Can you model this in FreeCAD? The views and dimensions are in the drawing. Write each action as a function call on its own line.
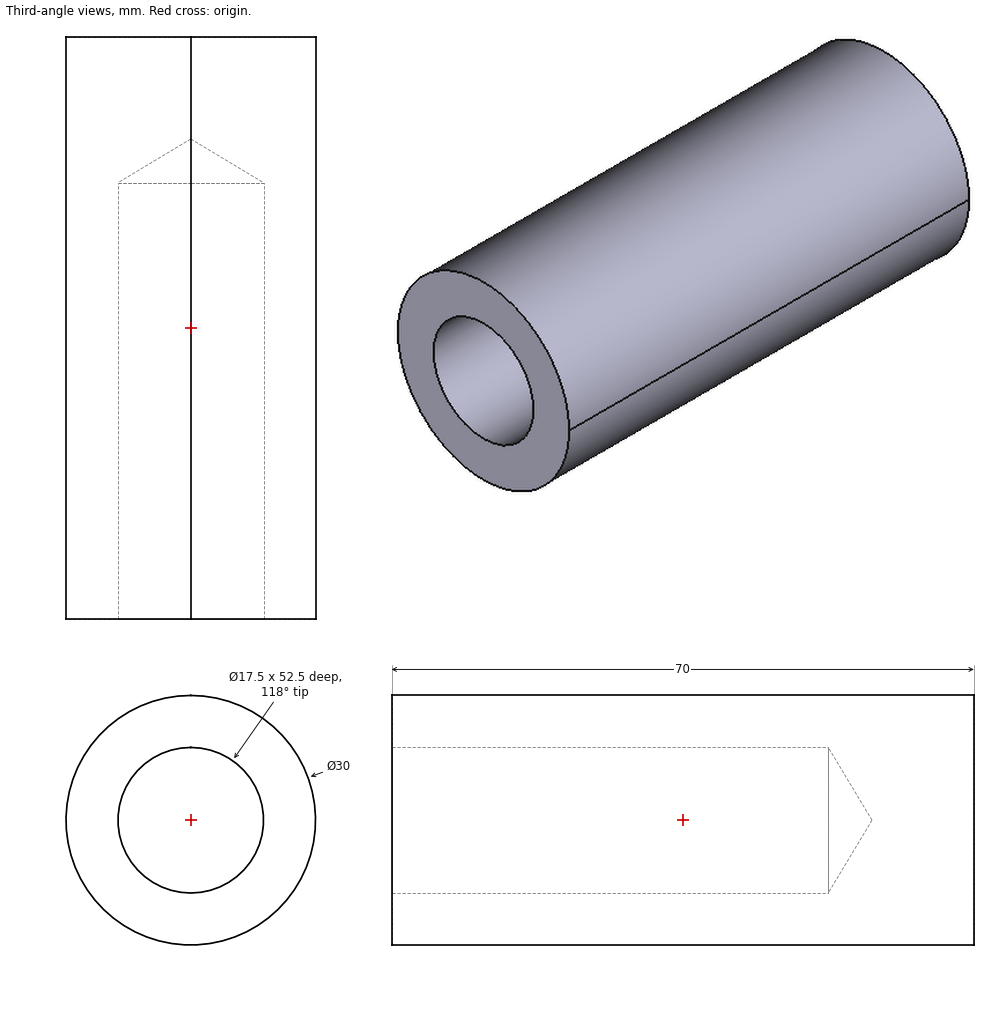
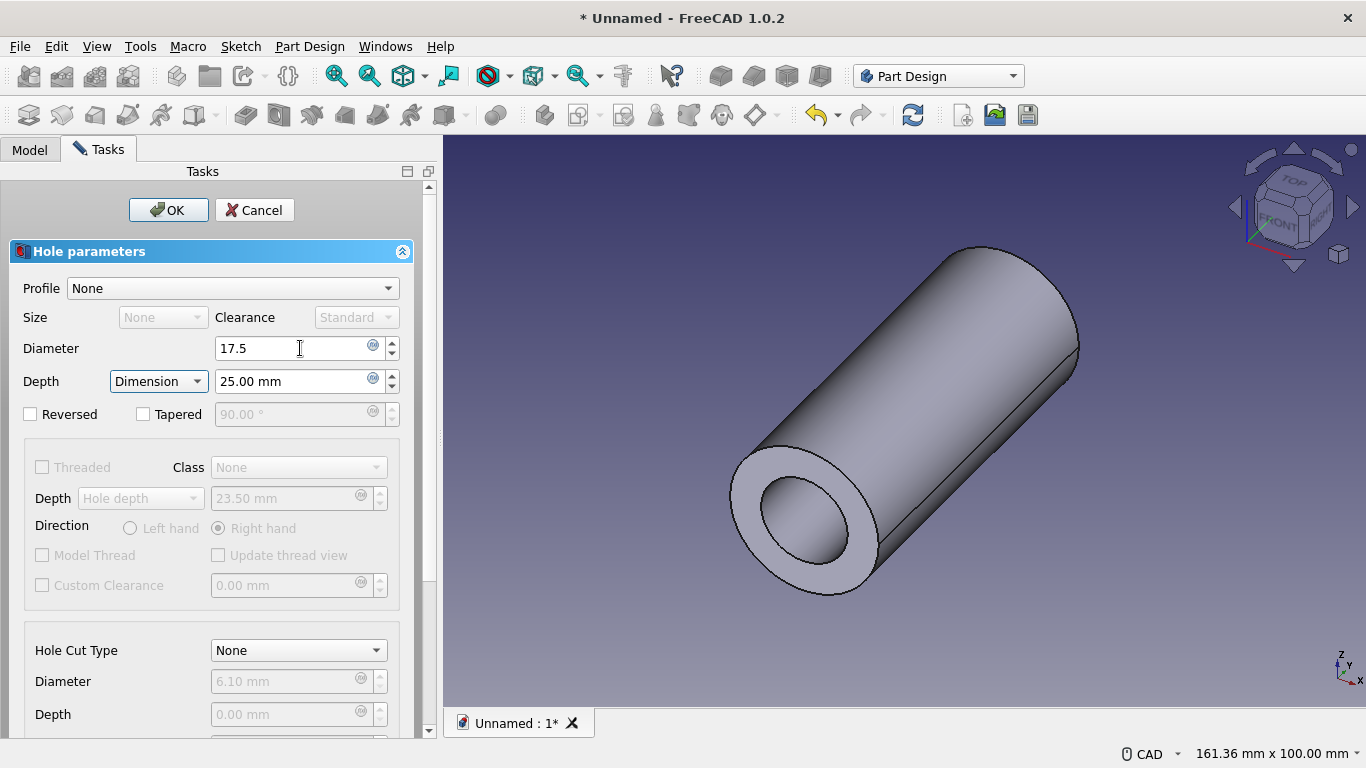
triple_click(300, 382)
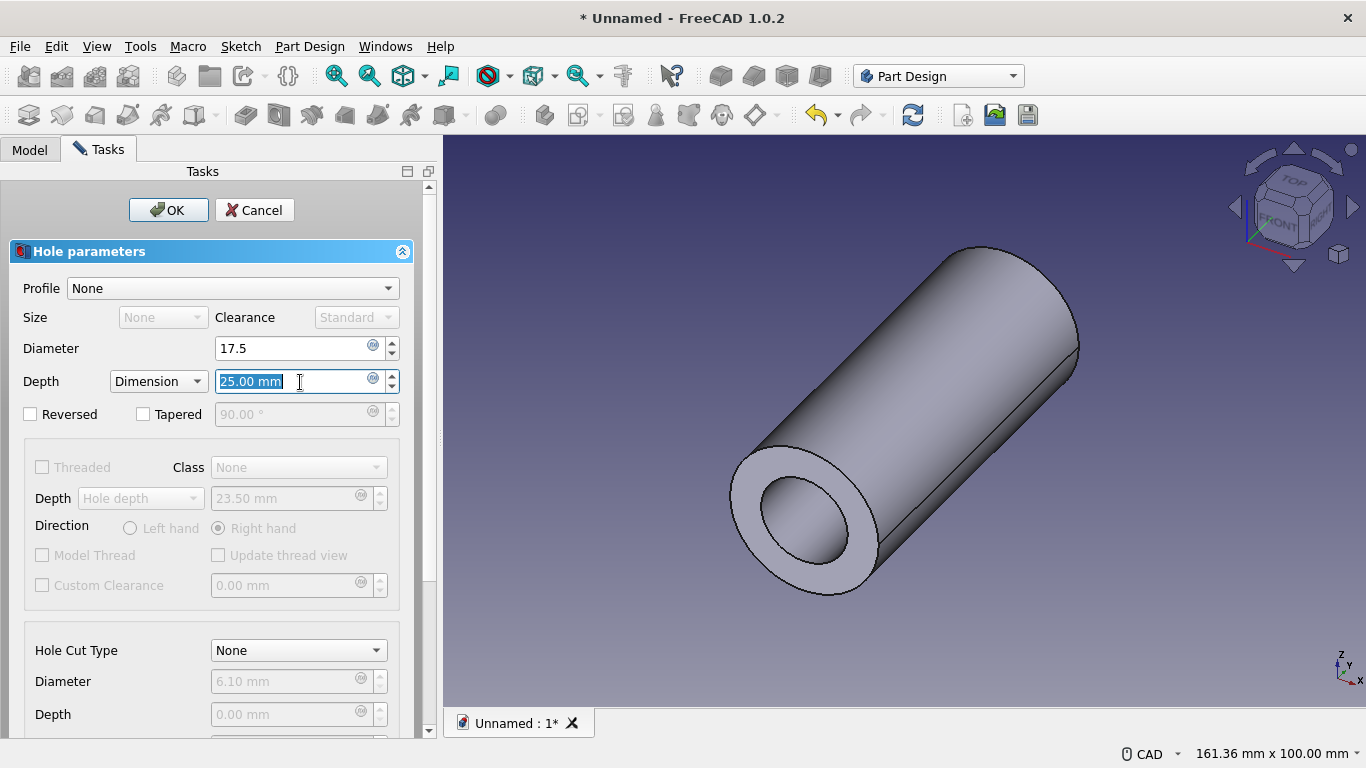
text(52.5)
key(Tab)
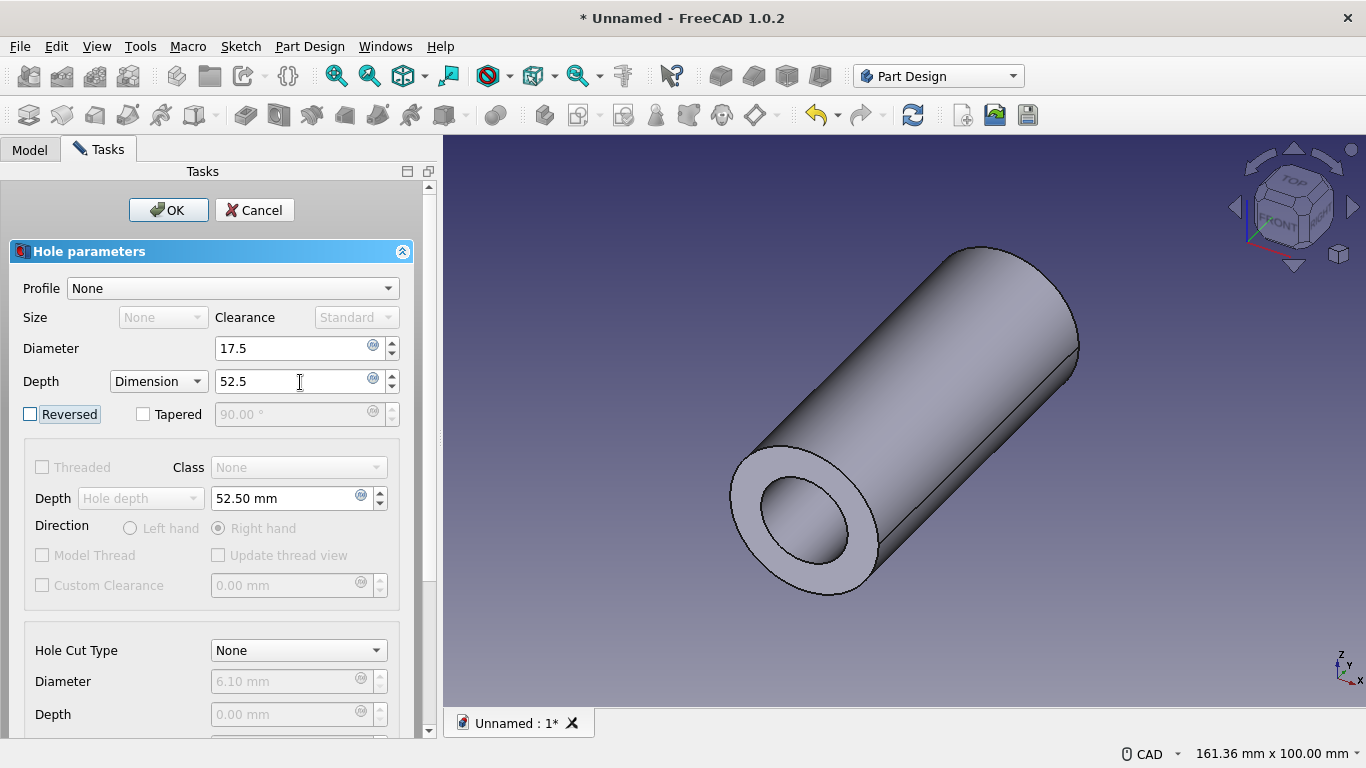
click(169, 210)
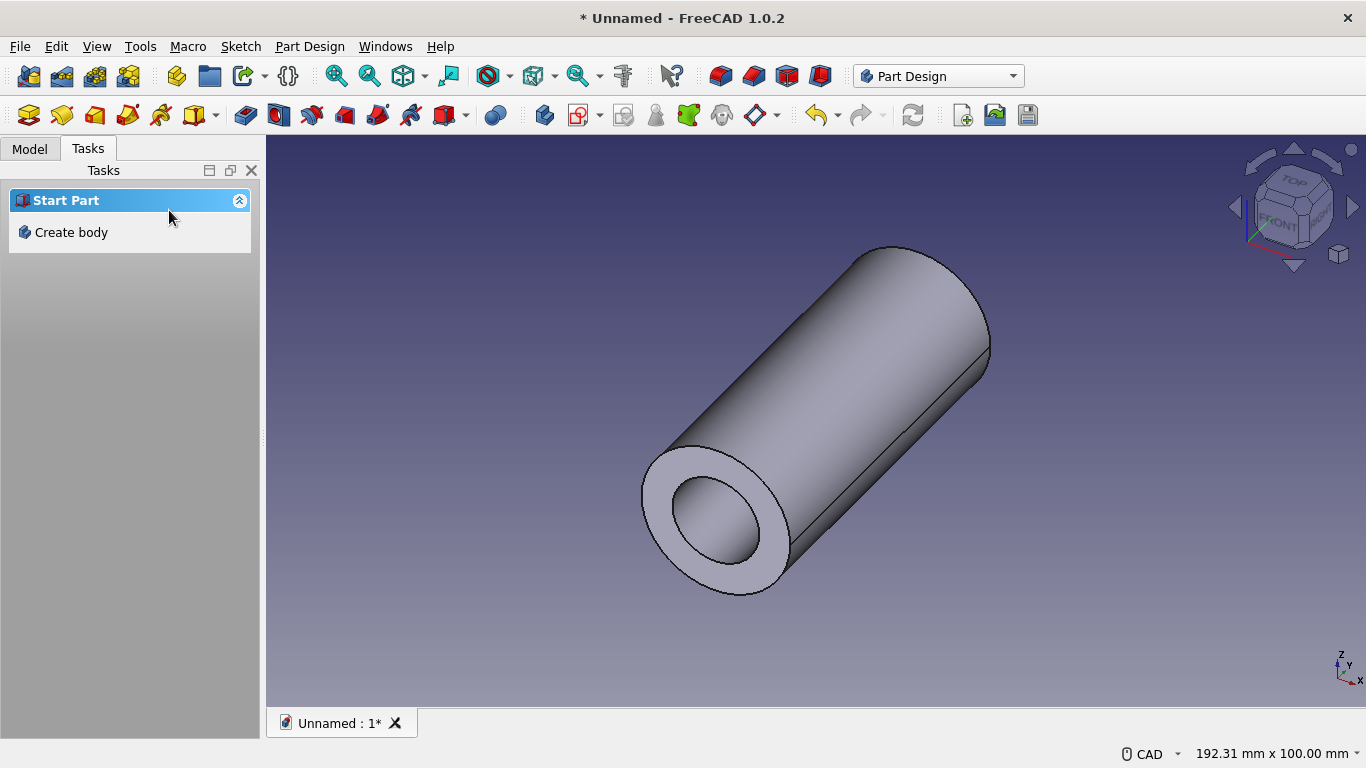
key(0)